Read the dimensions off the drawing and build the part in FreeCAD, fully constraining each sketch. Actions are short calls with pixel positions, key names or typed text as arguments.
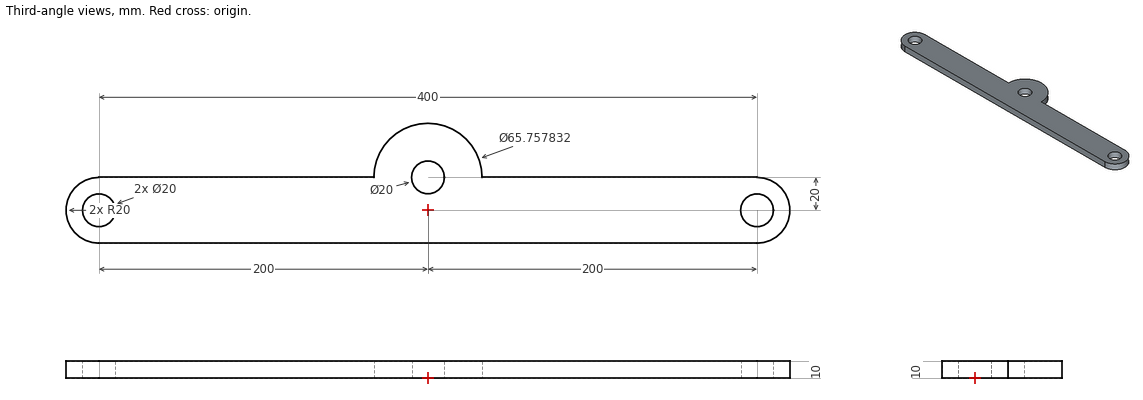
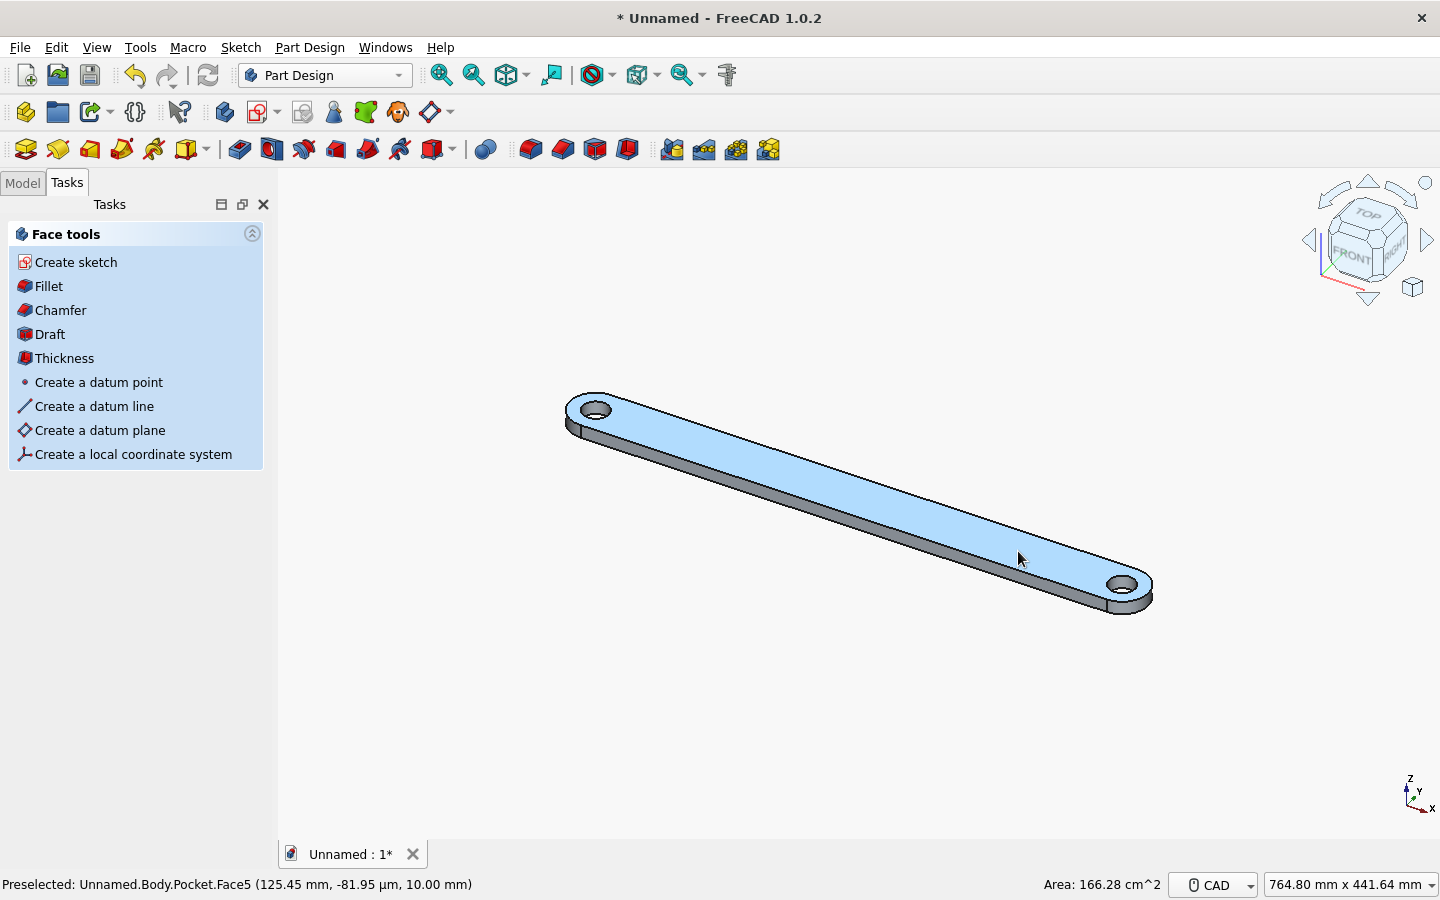
click(258, 112)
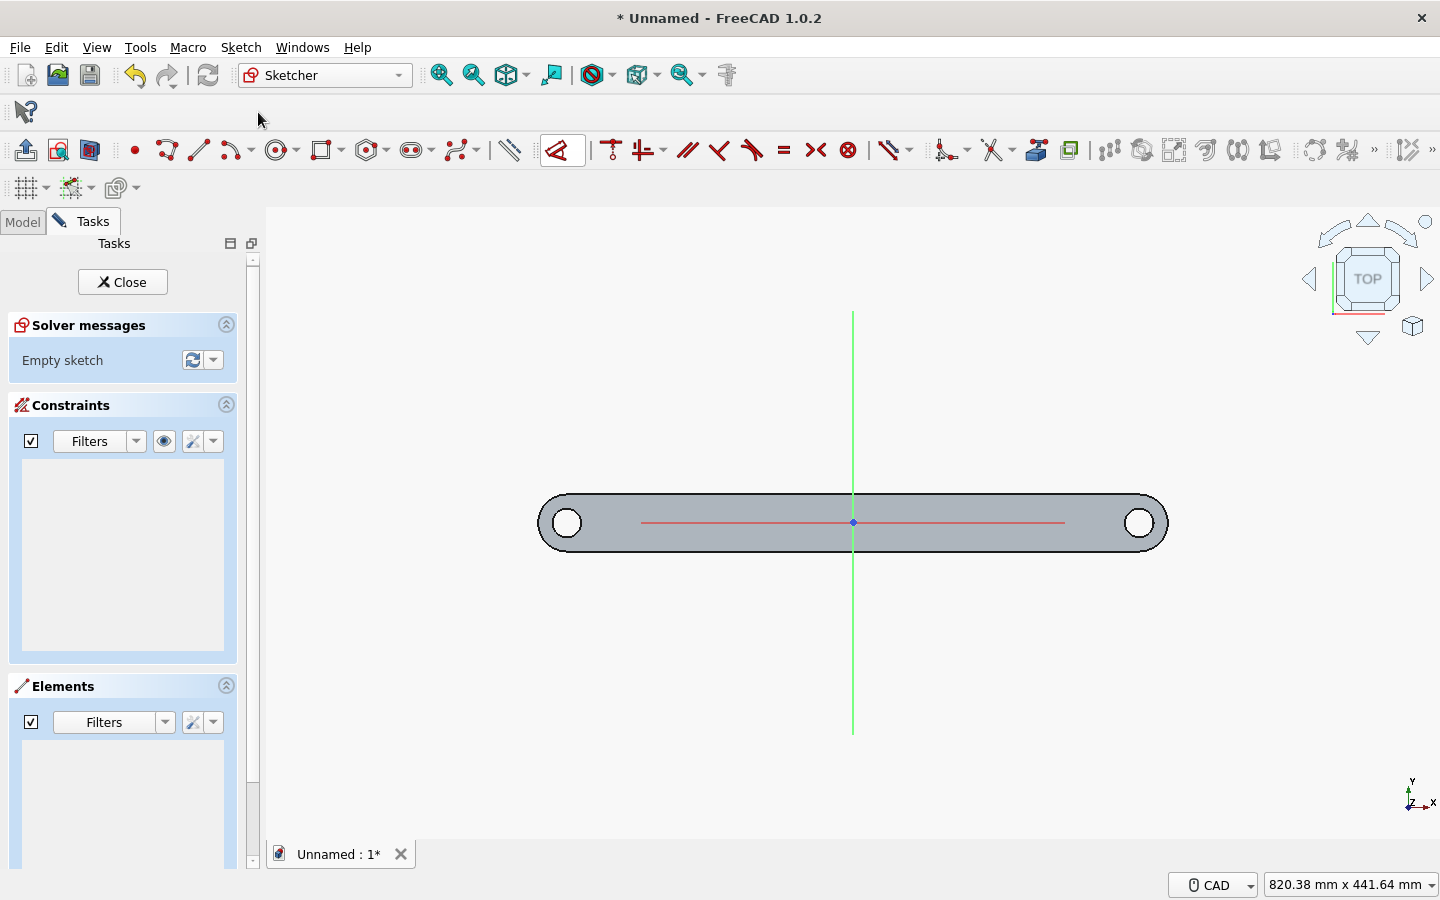
scroll(875, 485, up, 7)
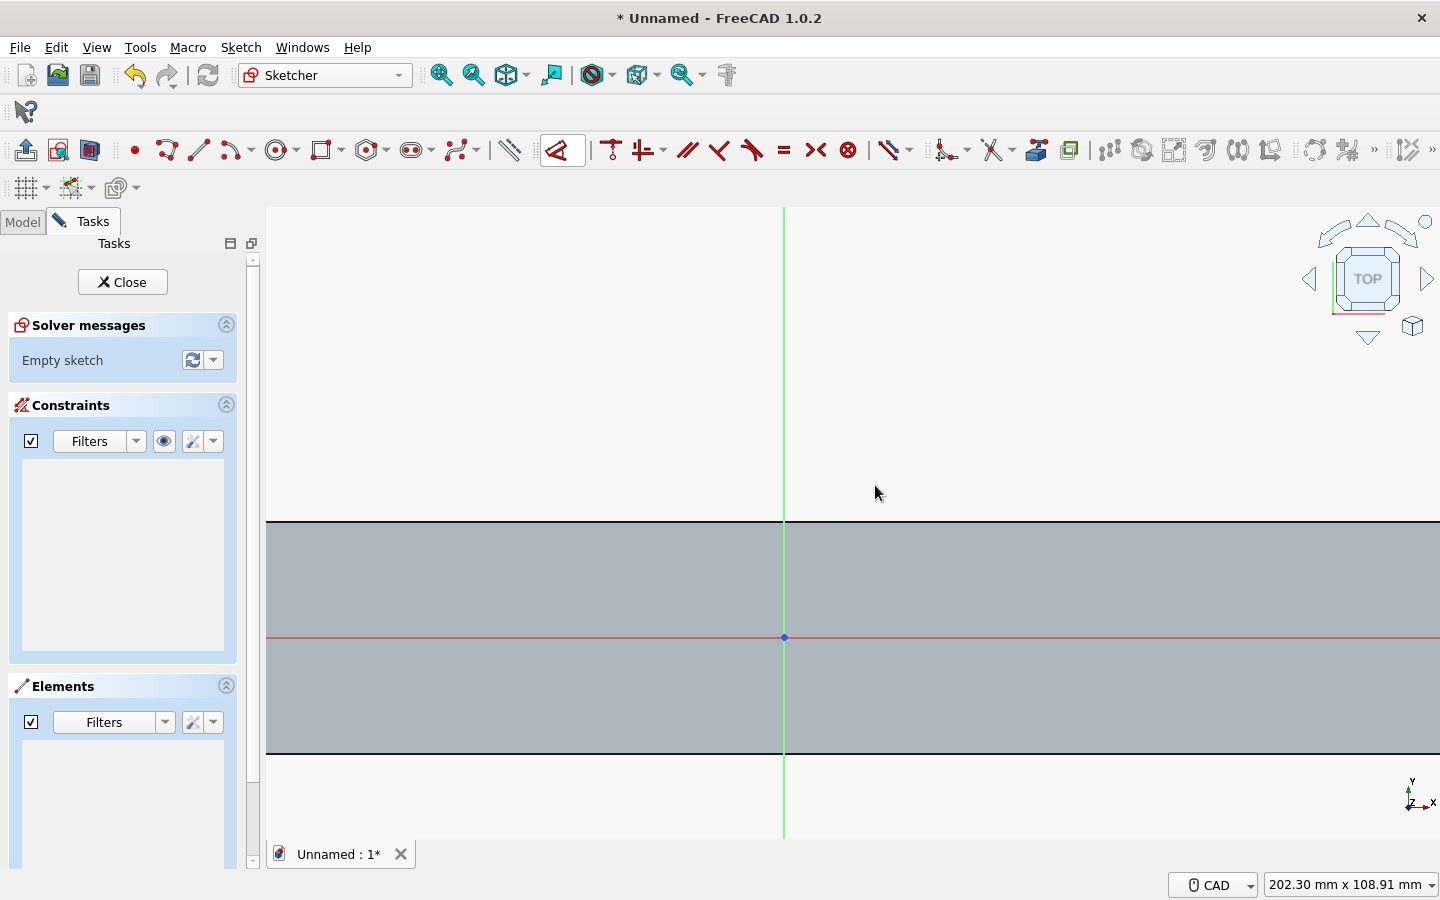
click(276, 150)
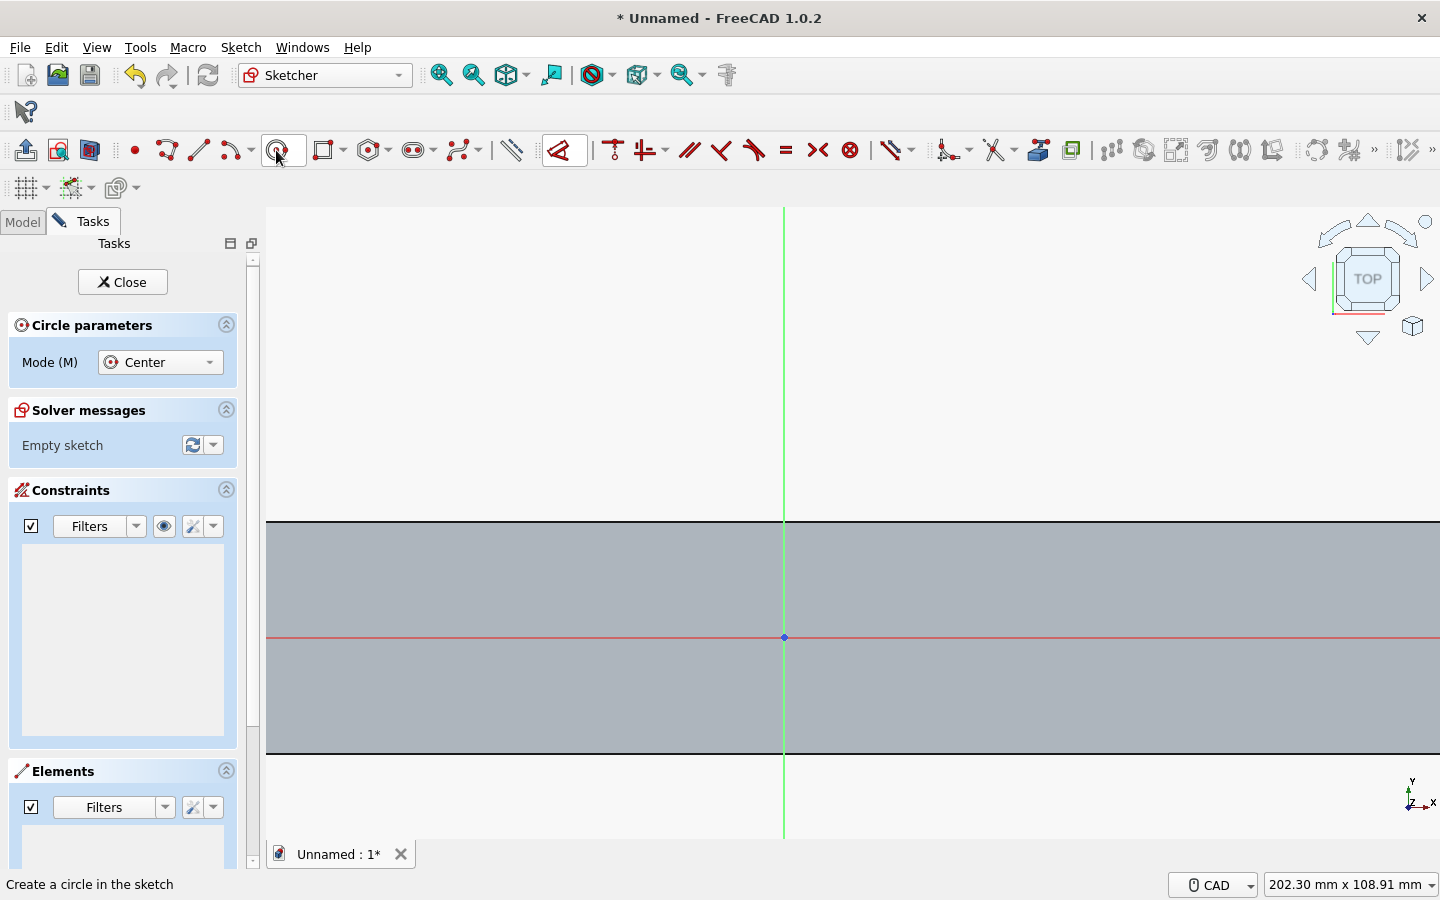
click(784, 522)
move(919, 387)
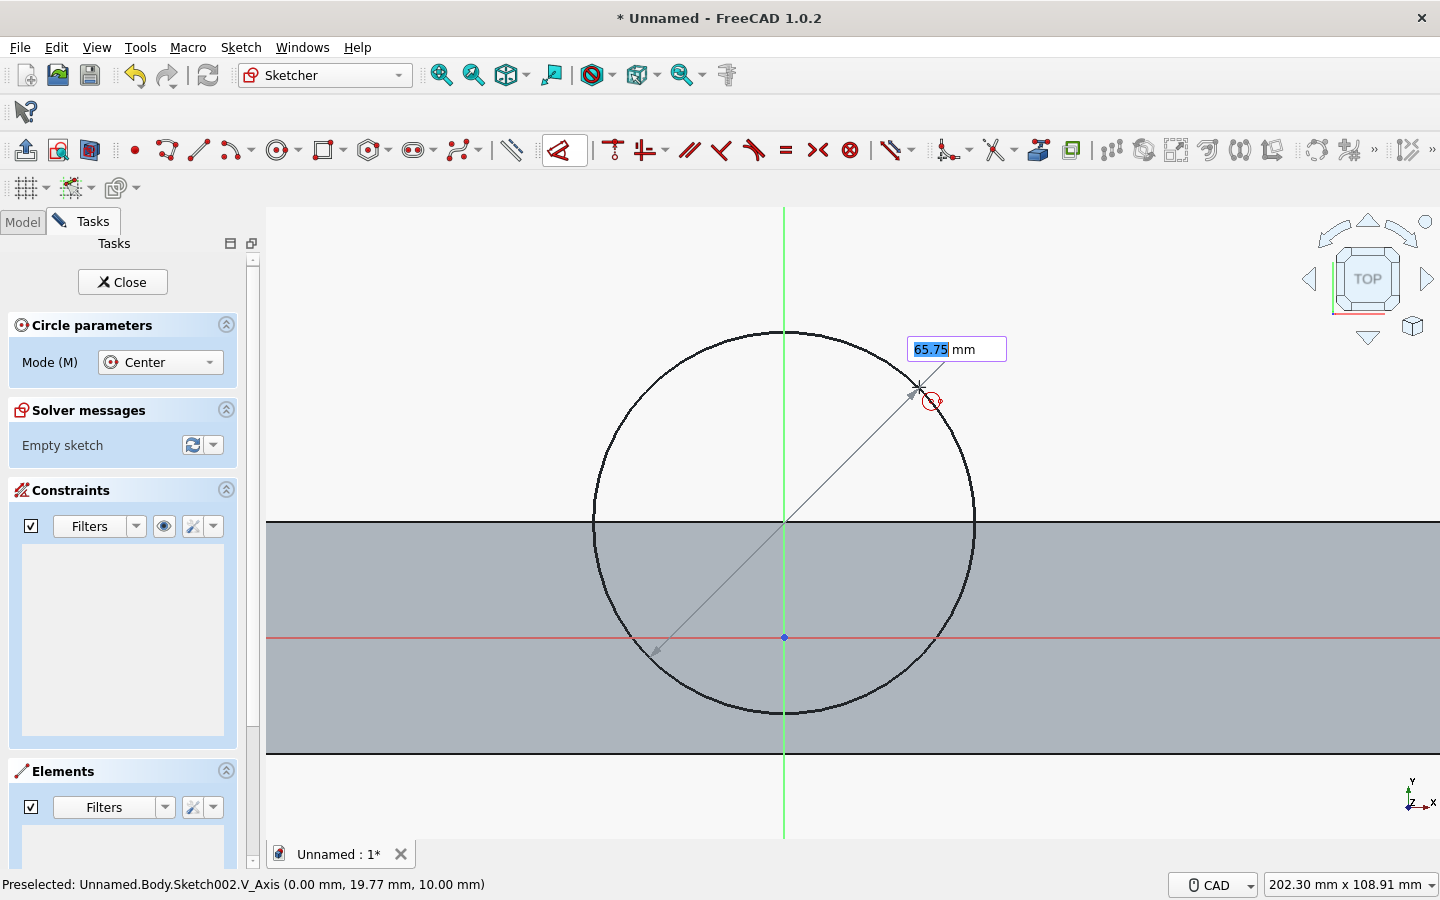
text(65.757832)
key(Return)
key(Escape)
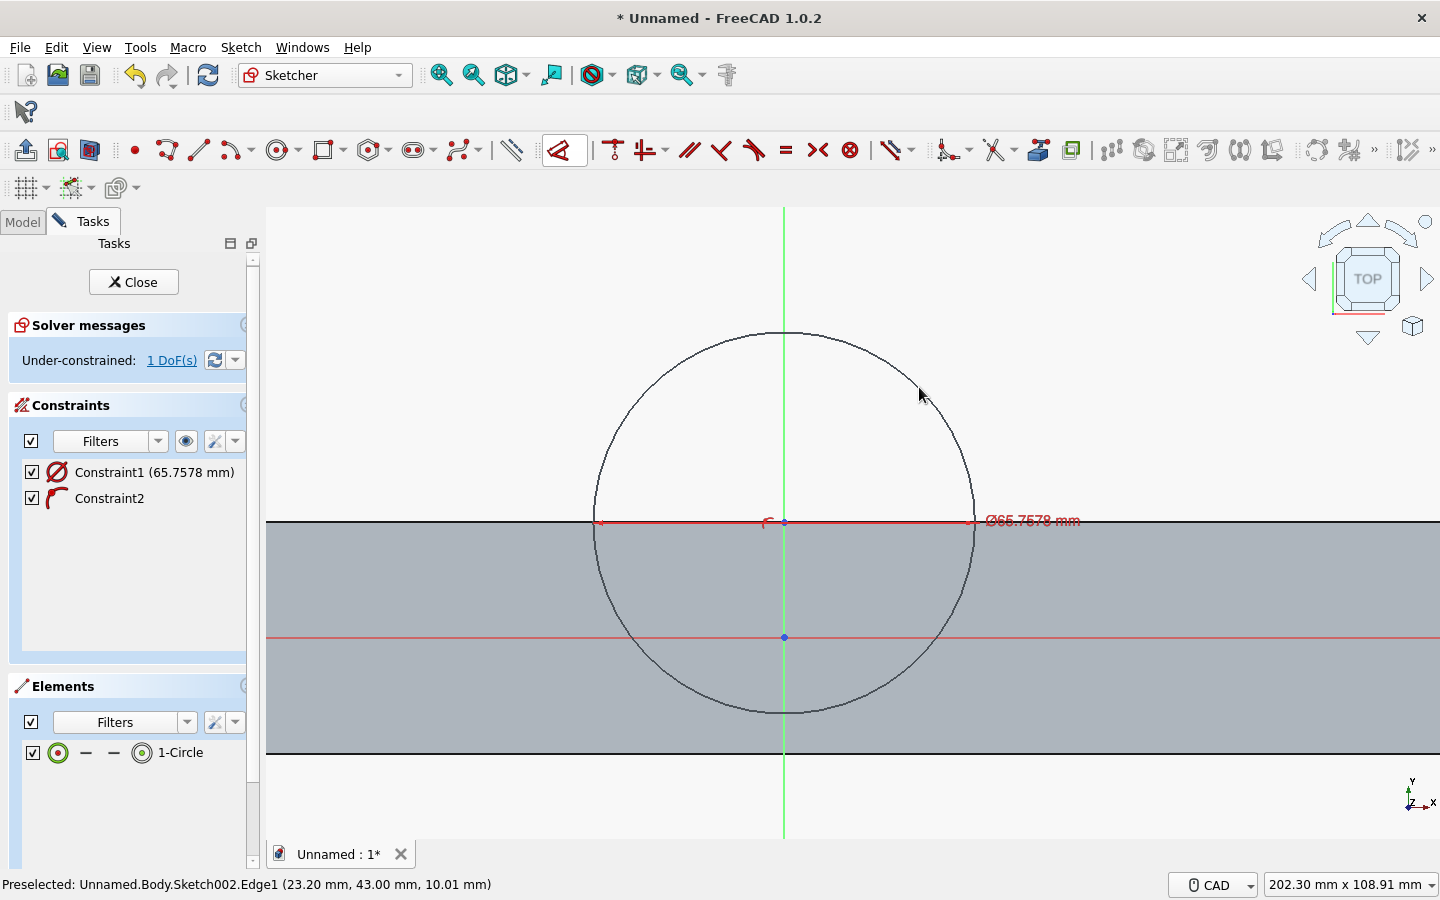
click(784, 523)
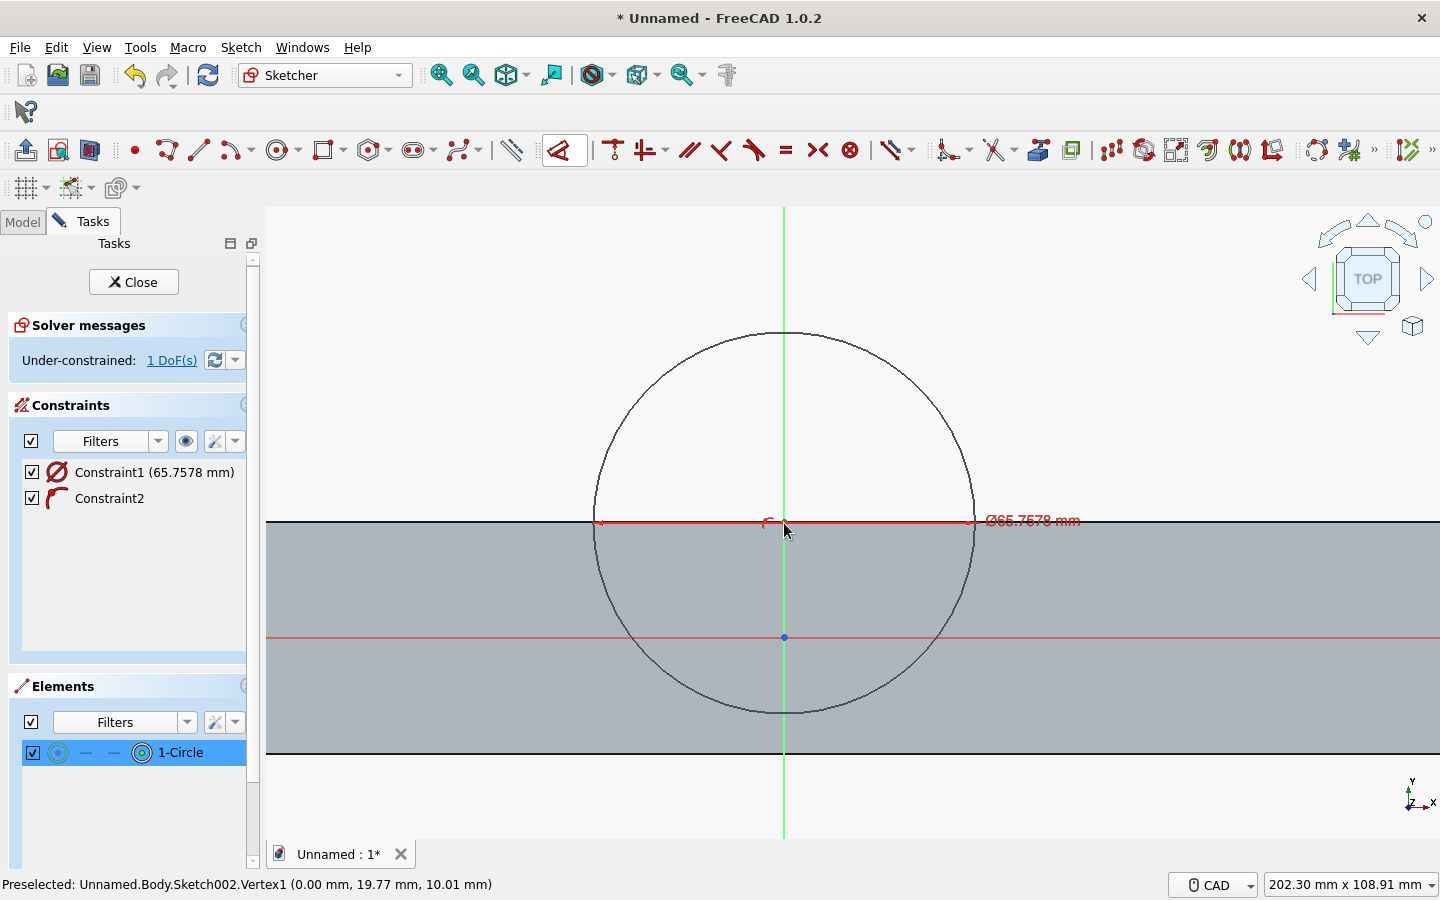
click(582, 150)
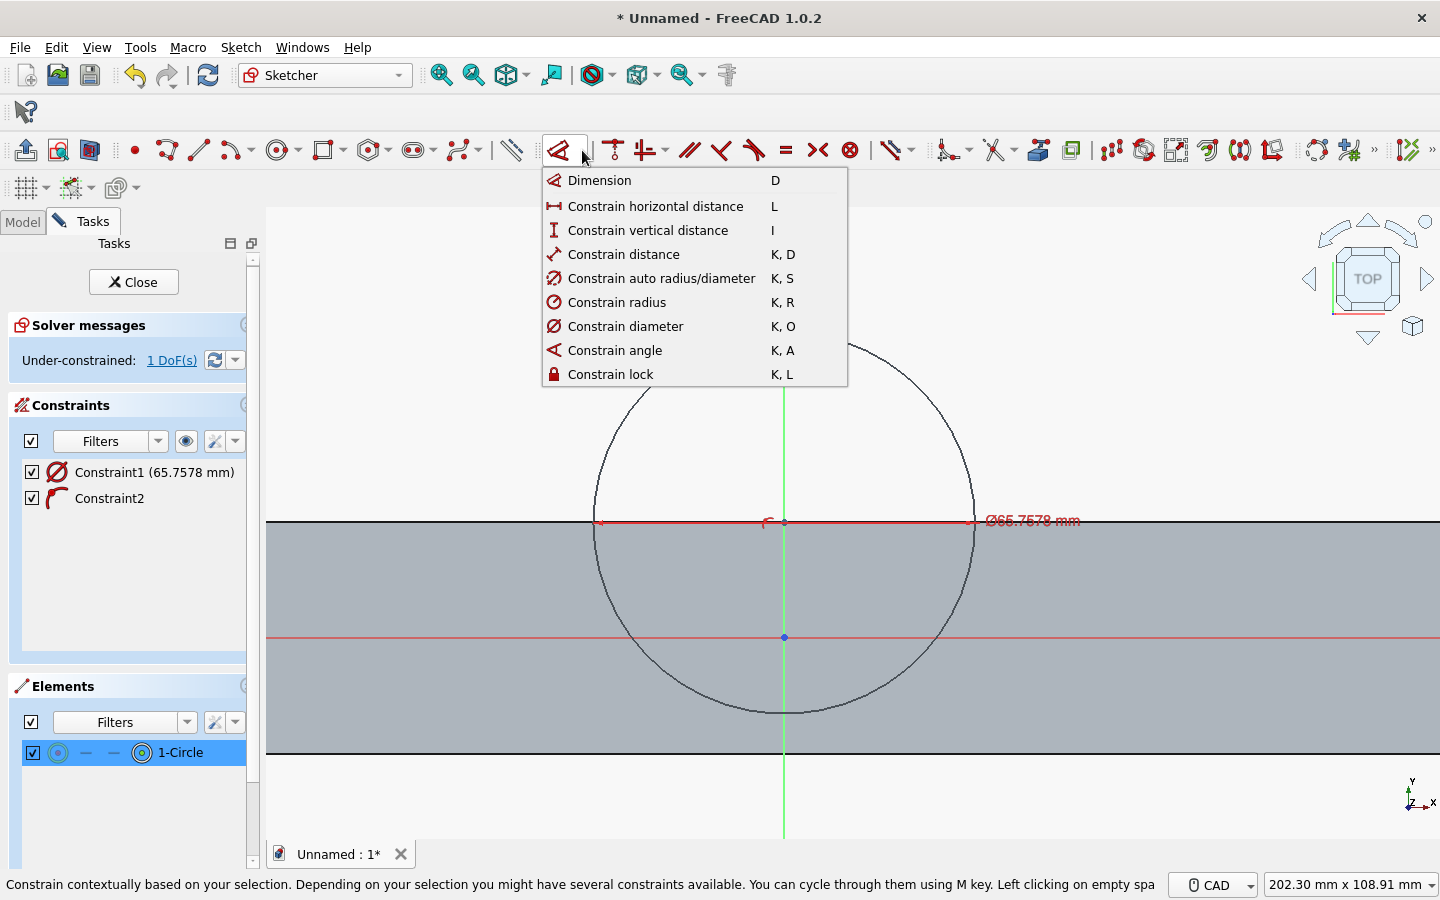
click(695, 230)